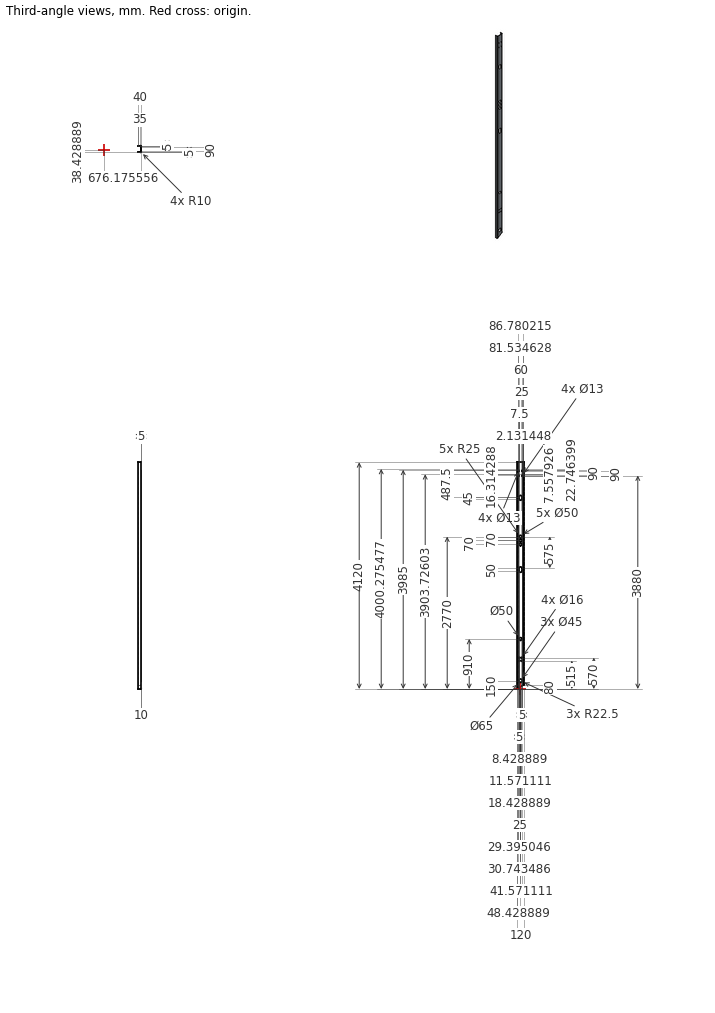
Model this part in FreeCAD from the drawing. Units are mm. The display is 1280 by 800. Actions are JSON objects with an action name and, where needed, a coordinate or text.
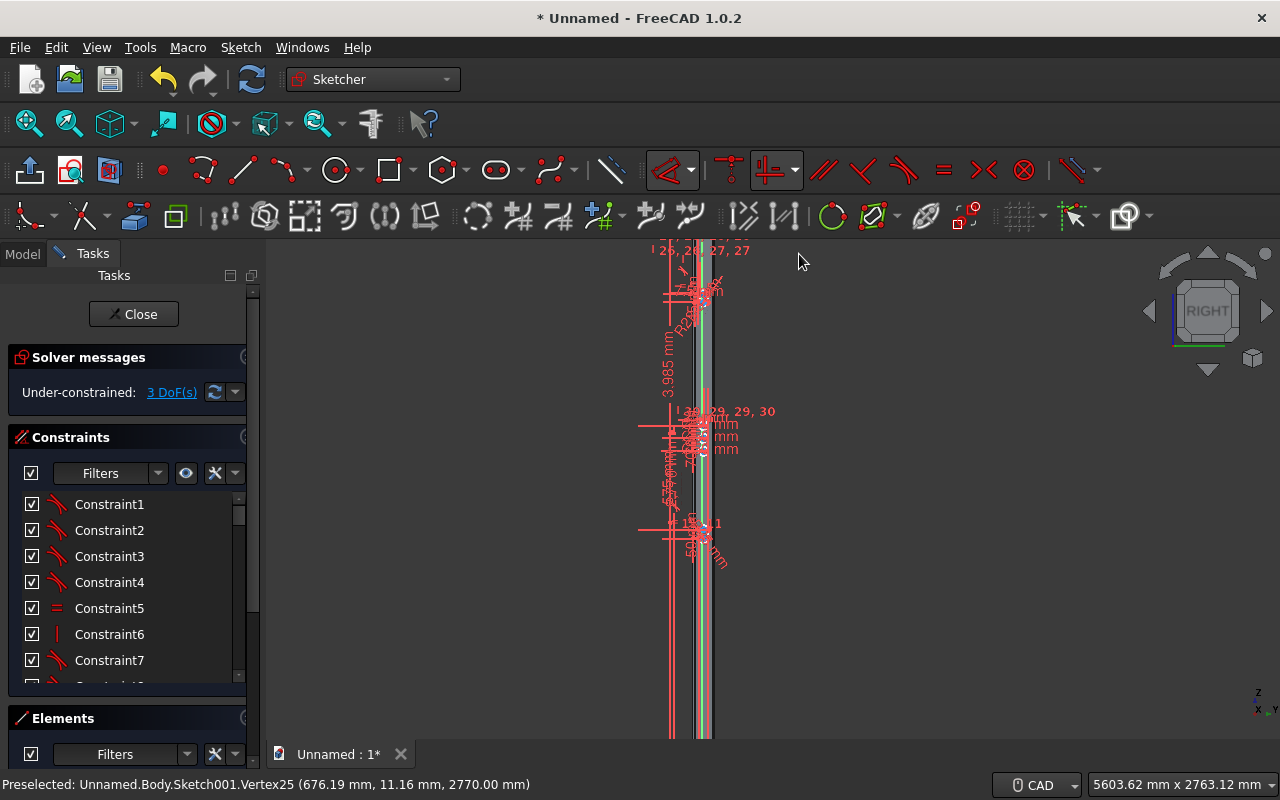
{"action": "scroll", "coordinate": [700, 294], "scroll_direction": "up", "scroll_amount": 6}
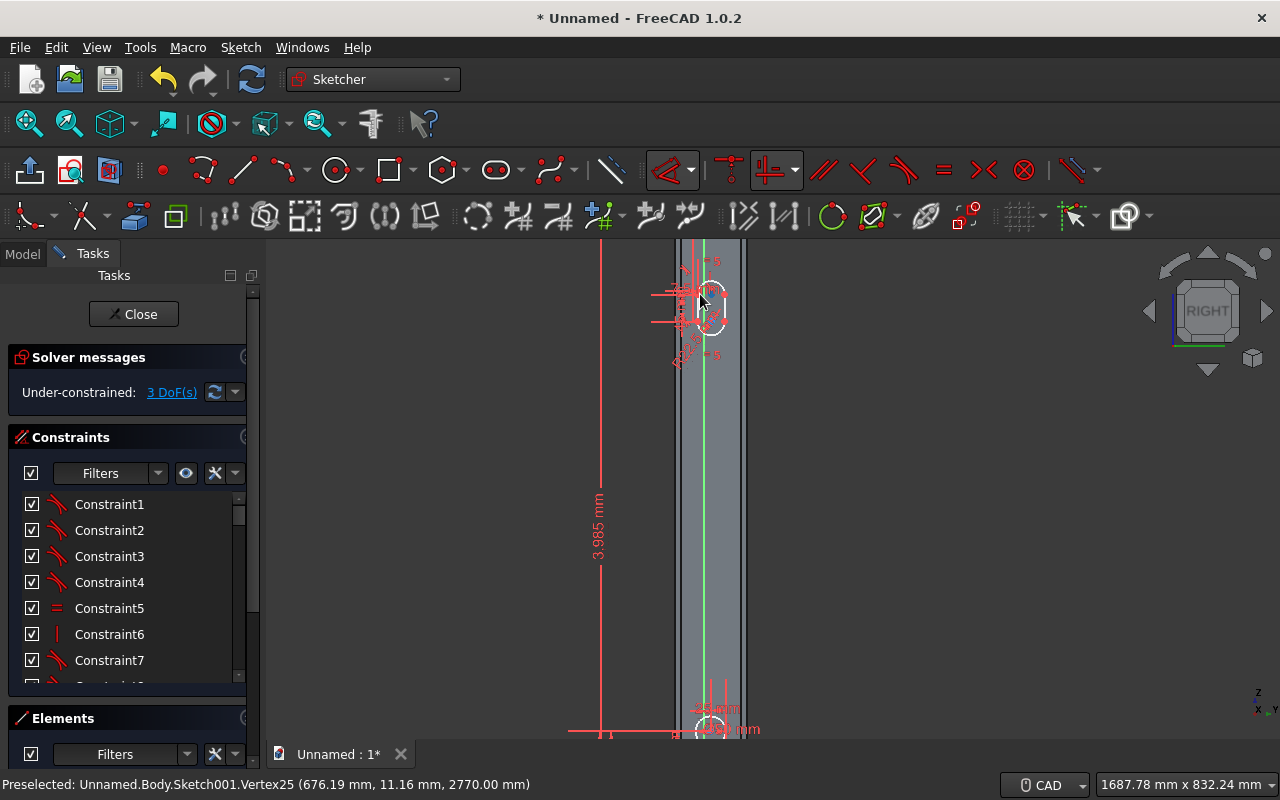
{"action": "left_click", "coordinate": [698, 295]}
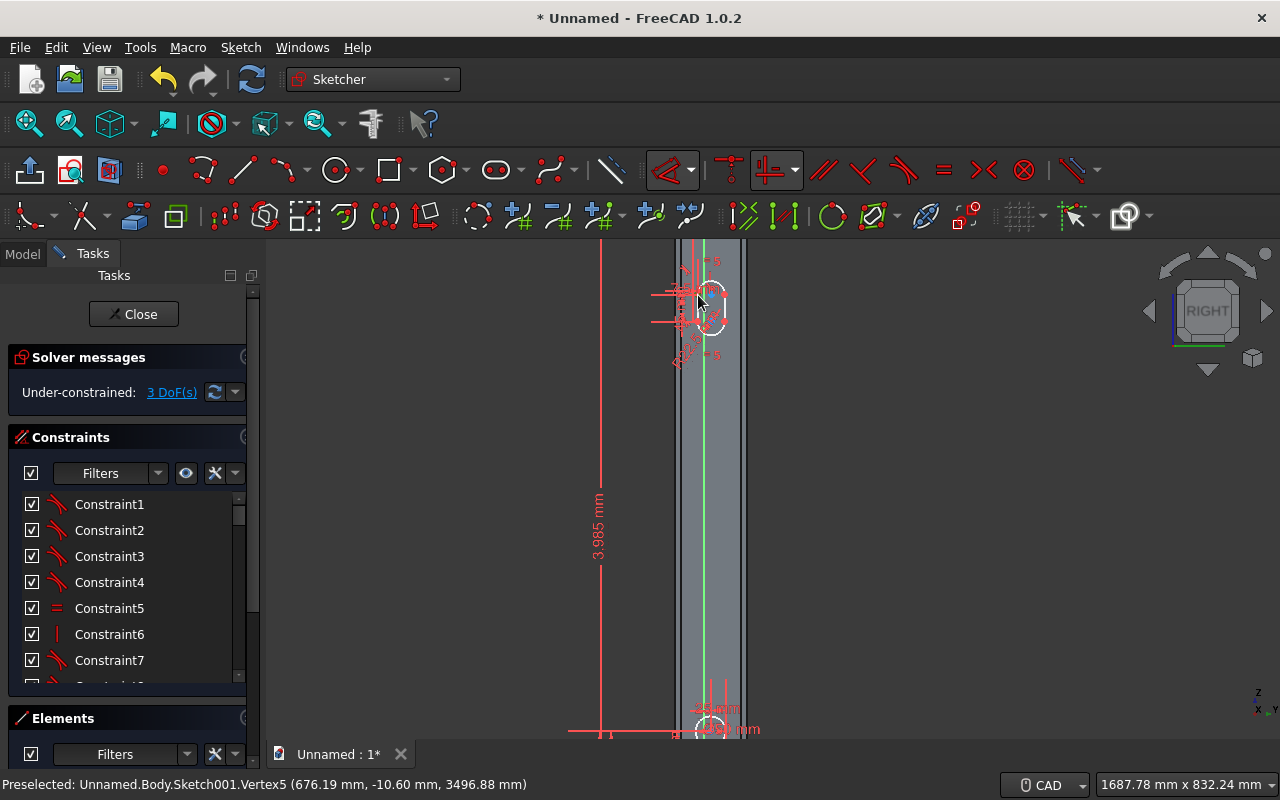
{"action": "scroll", "coordinate": [703, 378], "scroll_direction": "down", "scroll_amount": 10}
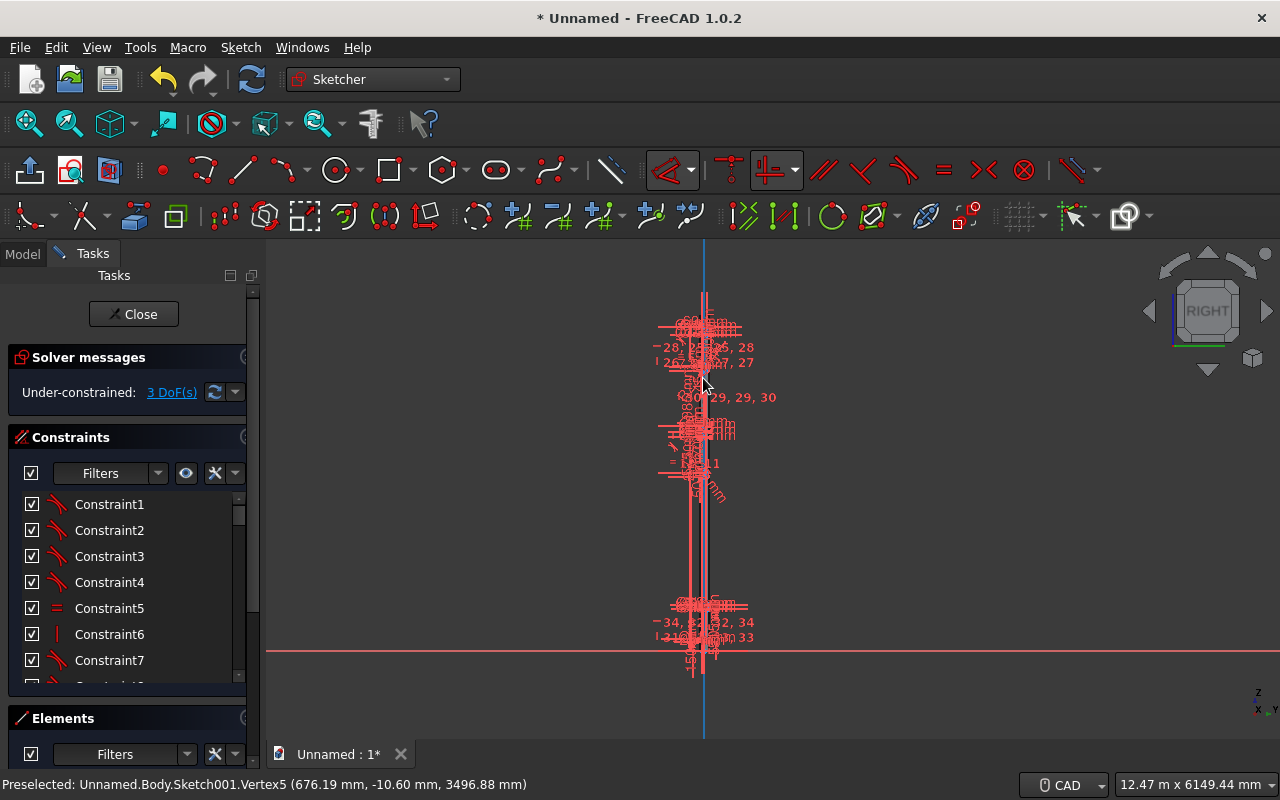
{"action": "scroll", "coordinate": [702, 327], "scroll_direction": "up", "scroll_amount": 5}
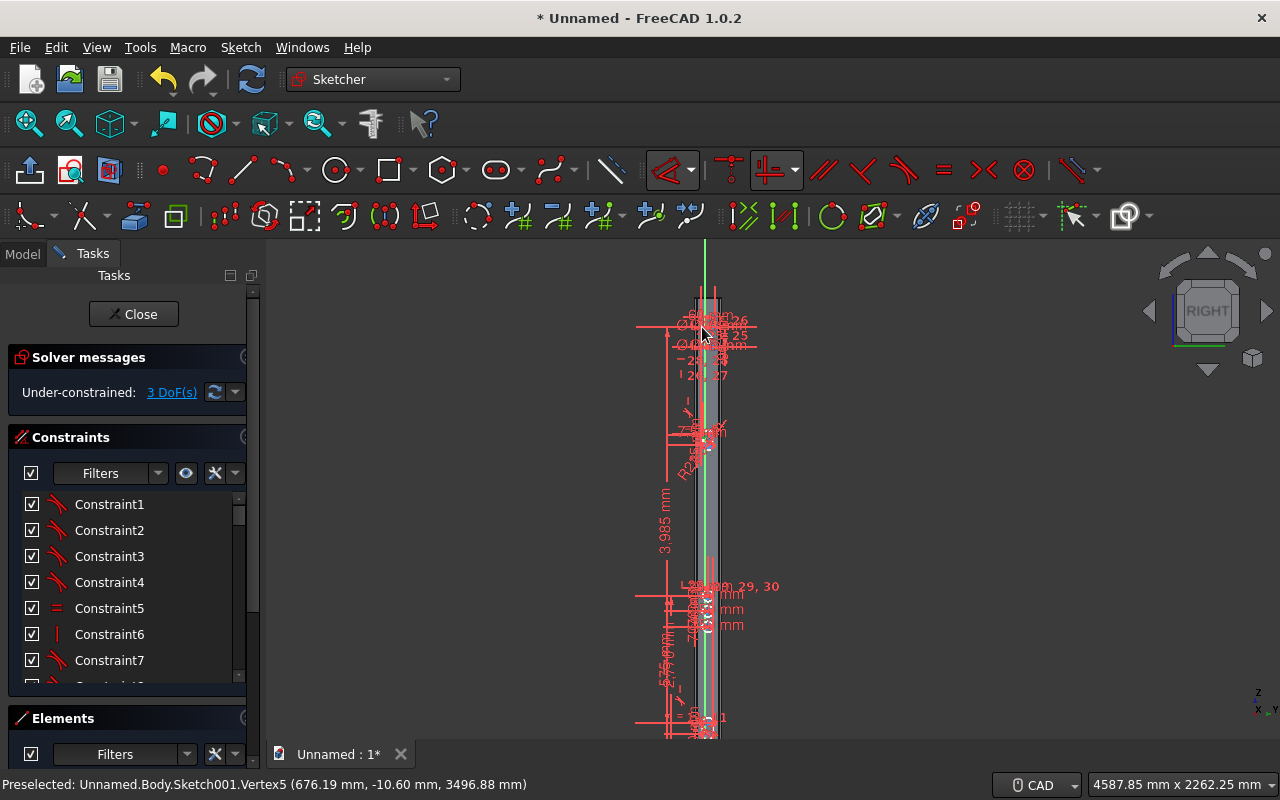
{"action": "left_click", "coordinate": [701, 327]}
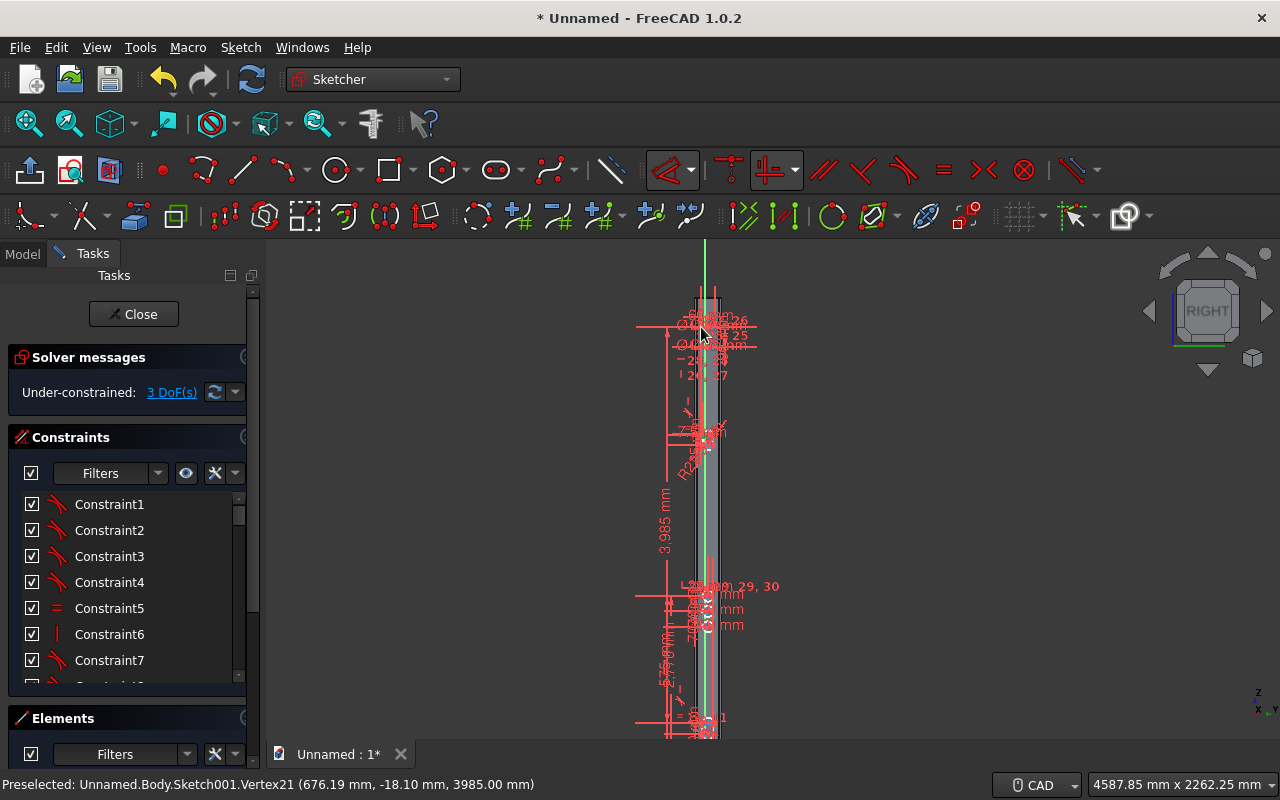
{"action": "left_click", "coordinate": [694, 170]}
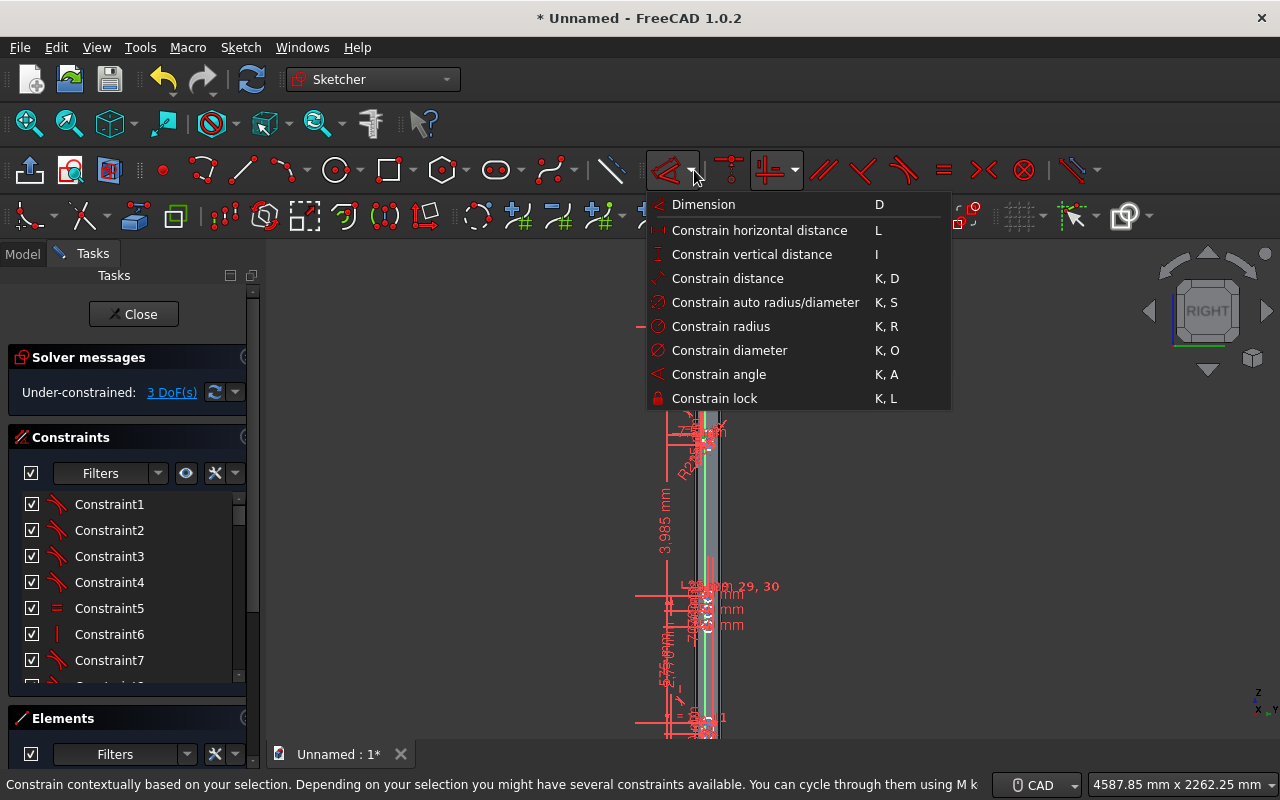
{"action": "left_click", "coordinate": [799, 254]}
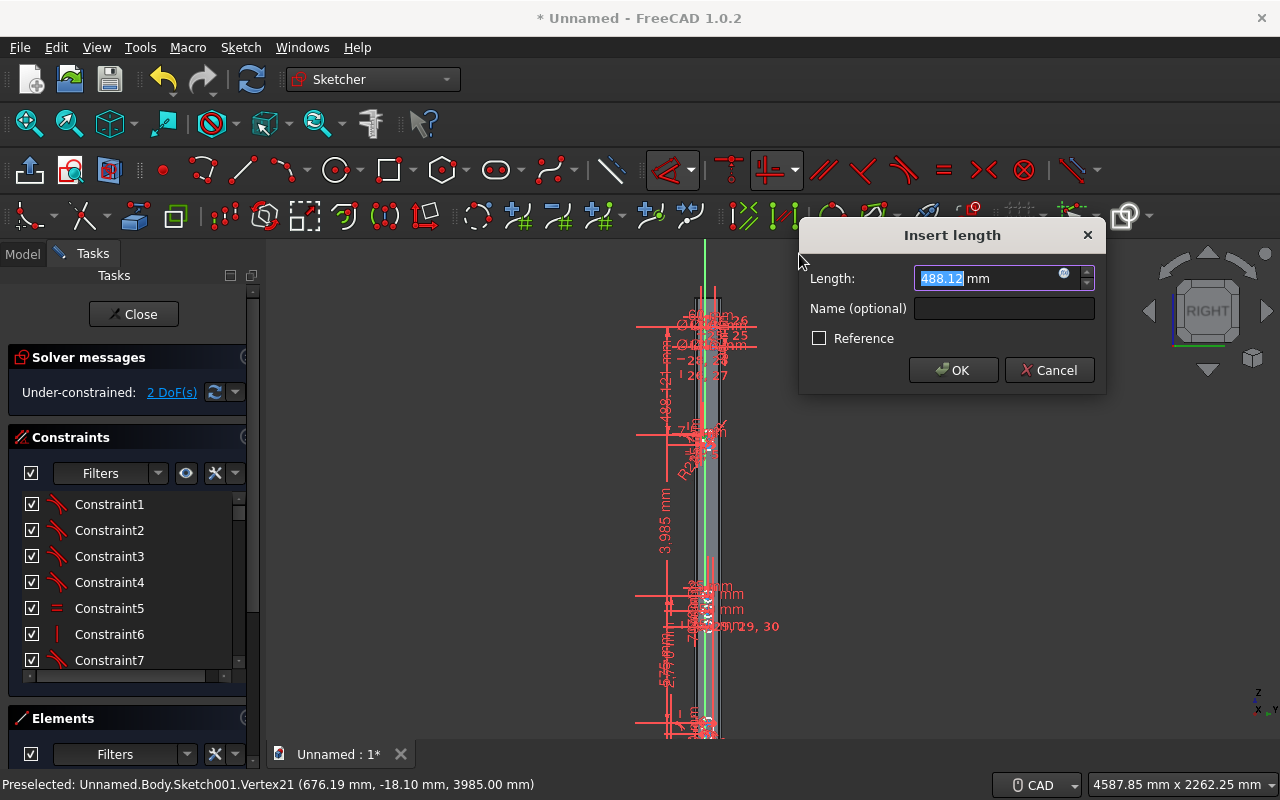
{"action": "type", "text": "487.5"}
{"action": "key", "text": "Return"}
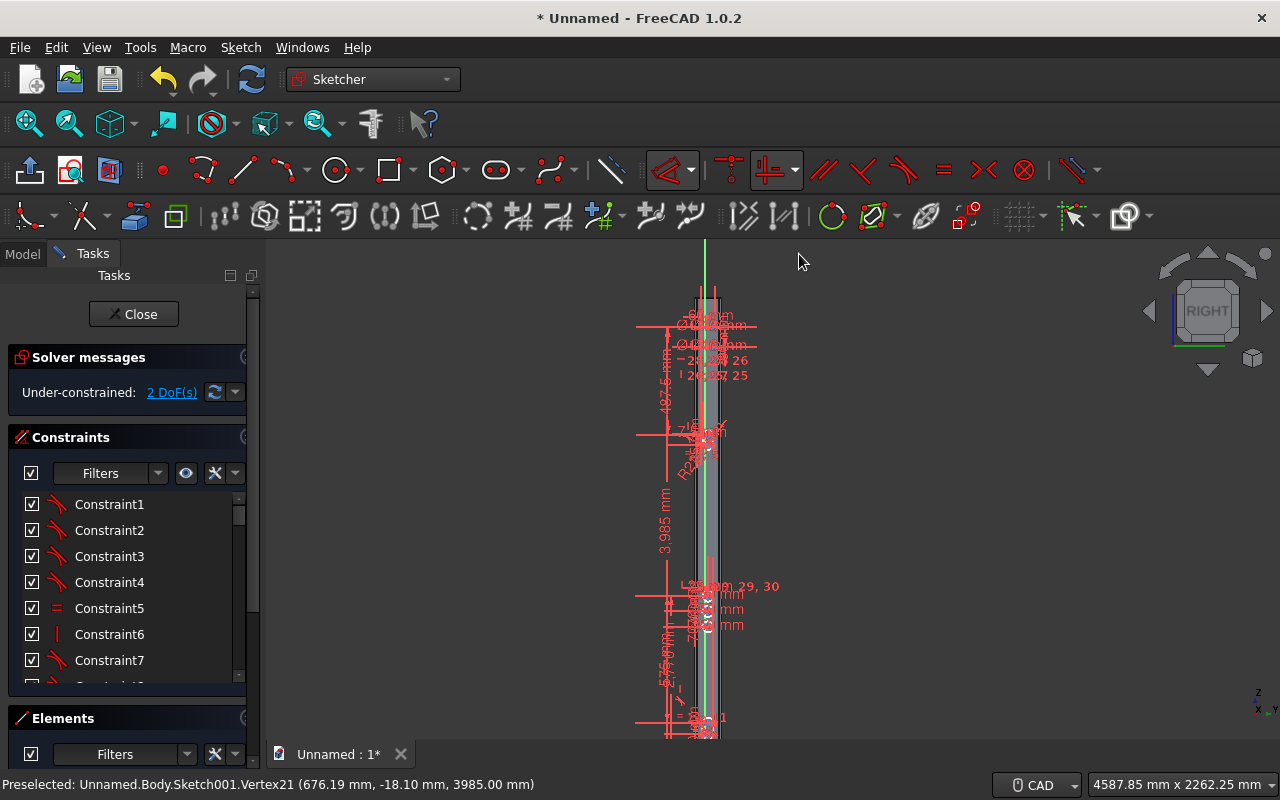
{"action": "scroll", "coordinate": [703, 327], "scroll_direction": "down", "scroll_amount": 5}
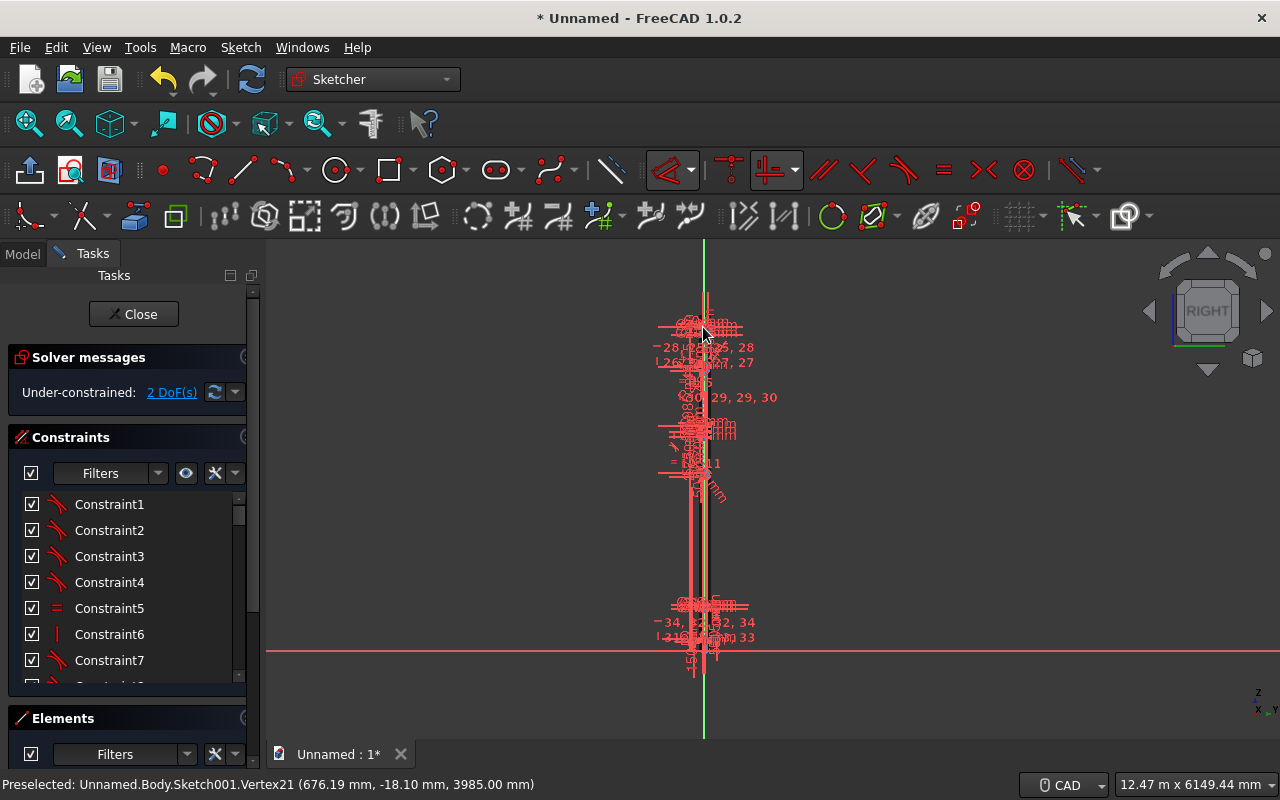
{"action": "scroll", "coordinate": [703, 605], "scroll_direction": "up", "scroll_amount": 21}